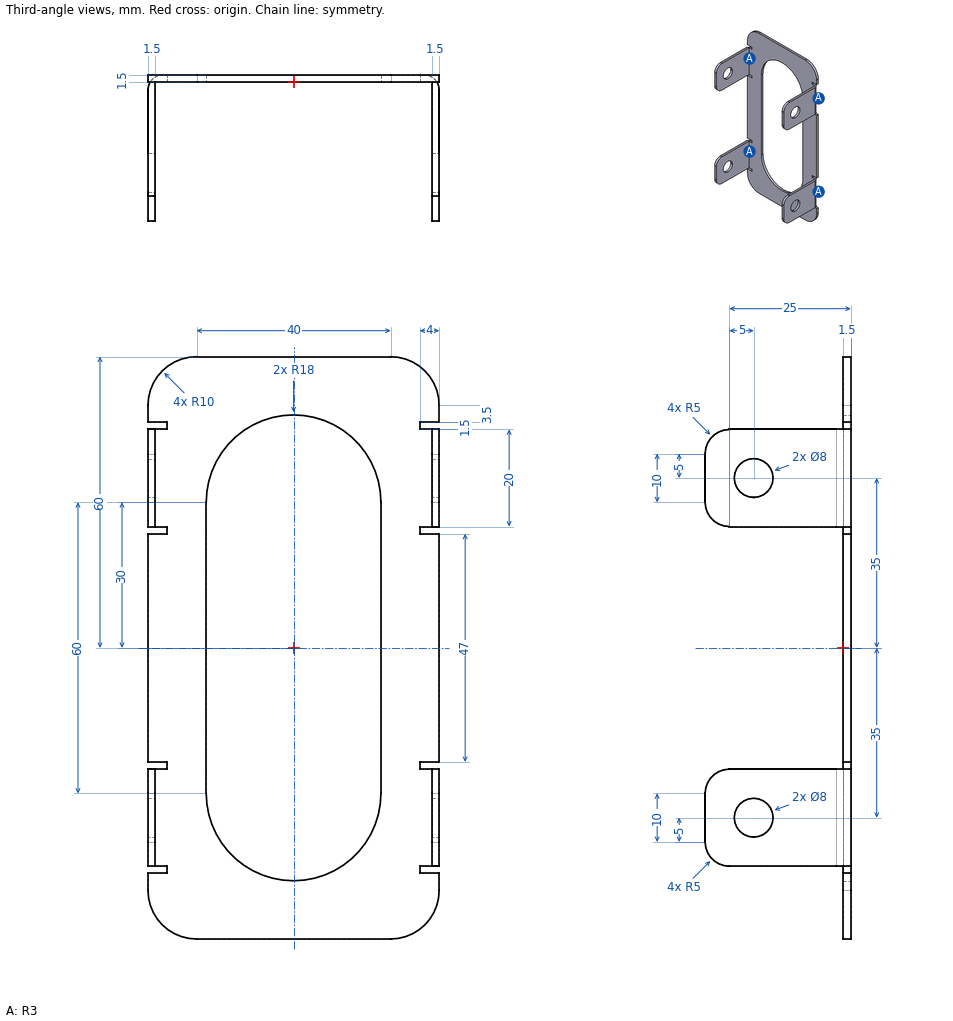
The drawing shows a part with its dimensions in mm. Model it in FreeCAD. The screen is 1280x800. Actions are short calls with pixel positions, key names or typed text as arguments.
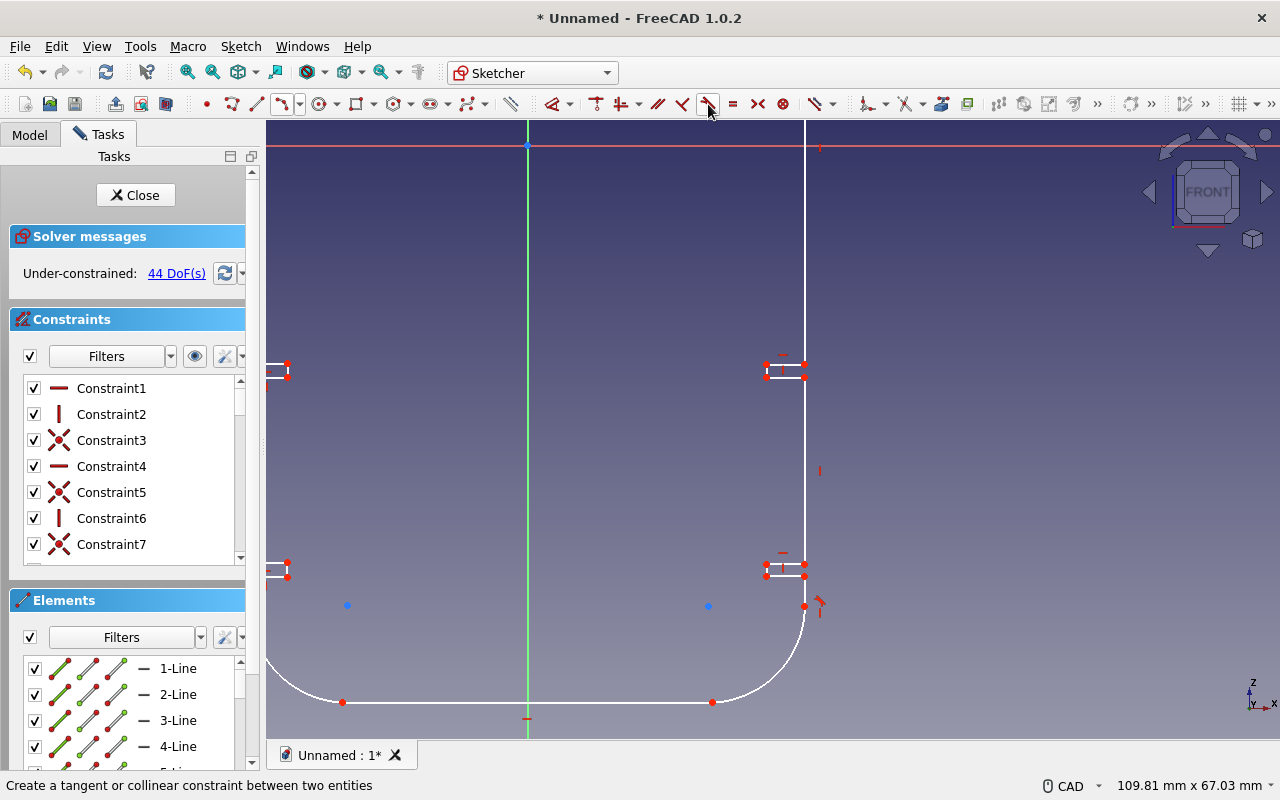
click(602, 703)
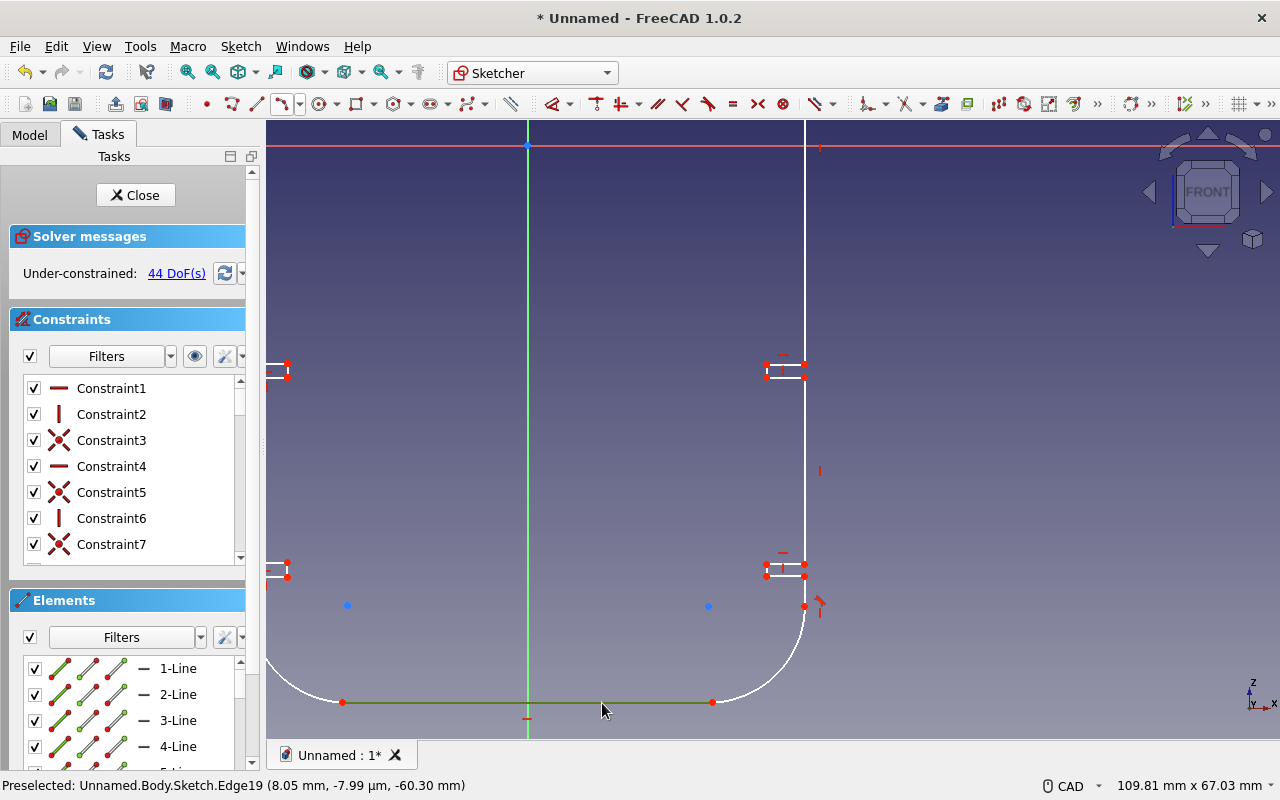
click(755, 691)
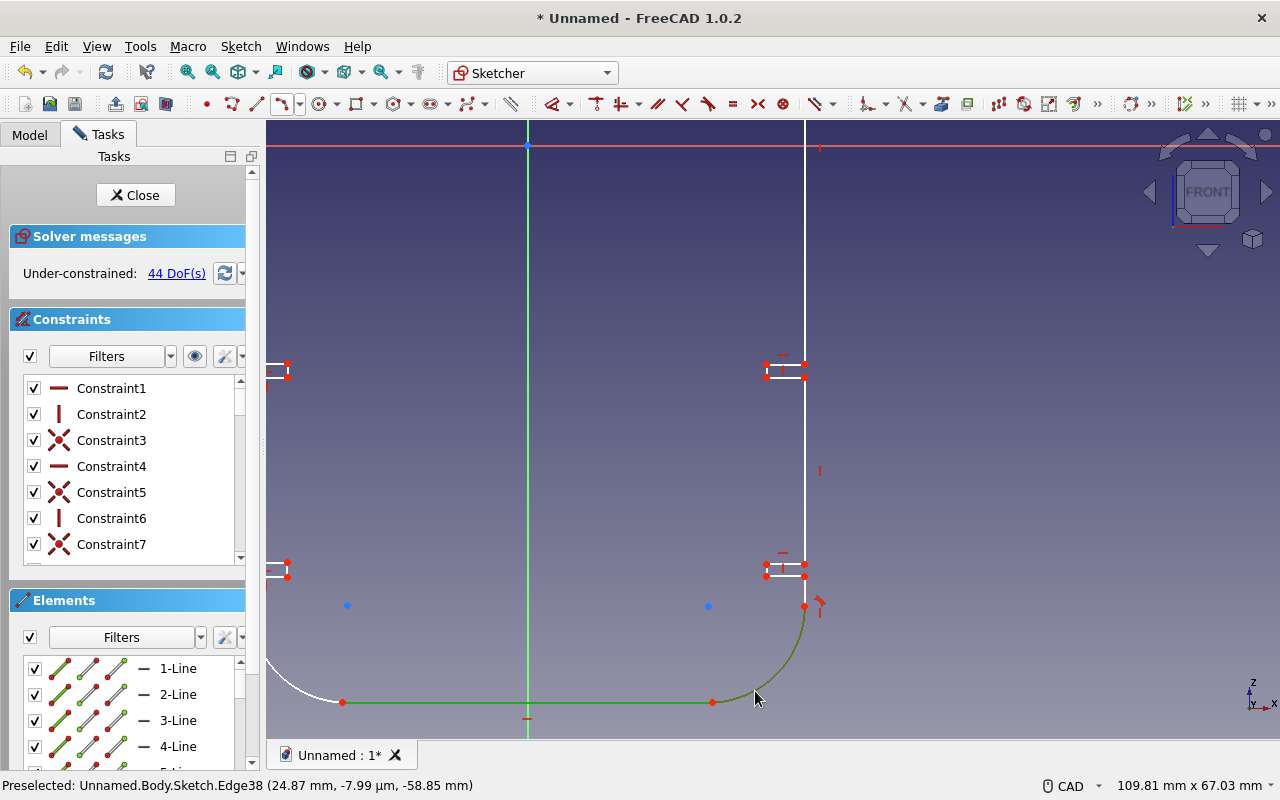
click(708, 104)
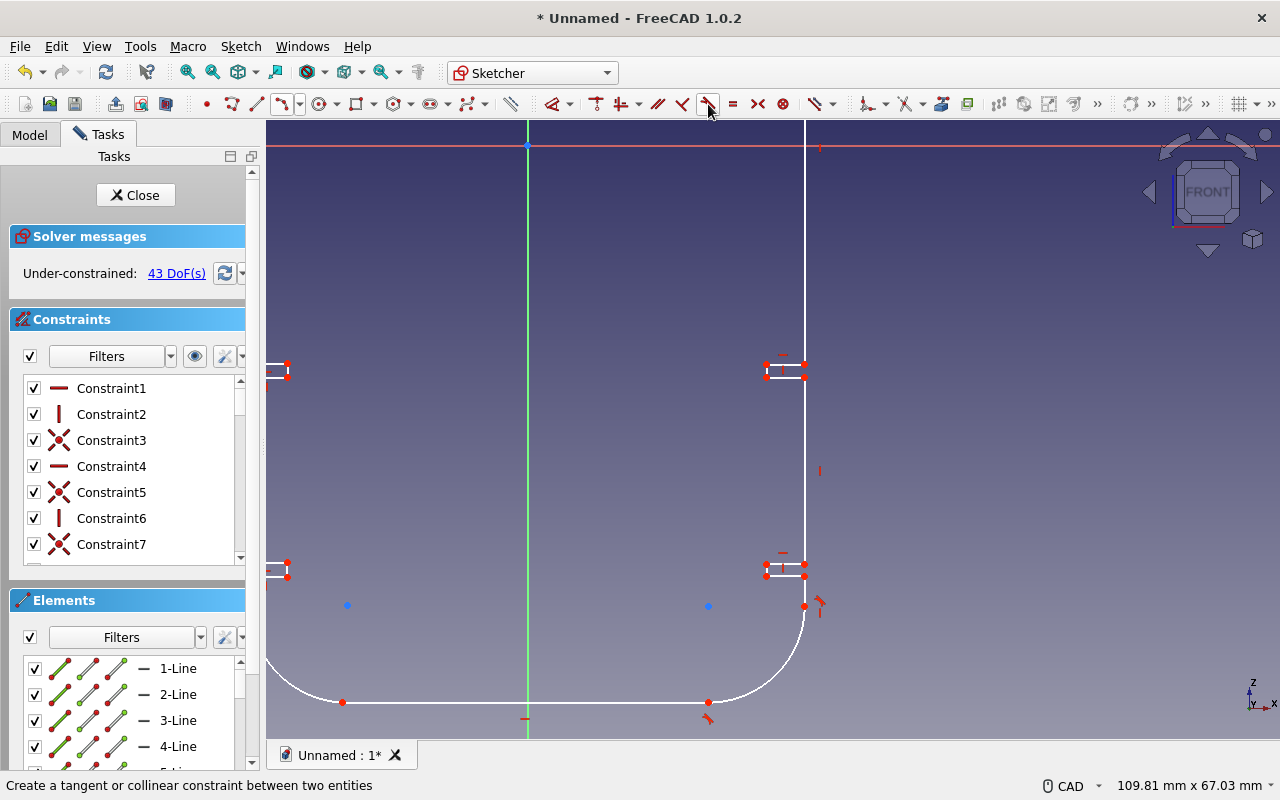
click(599, 703)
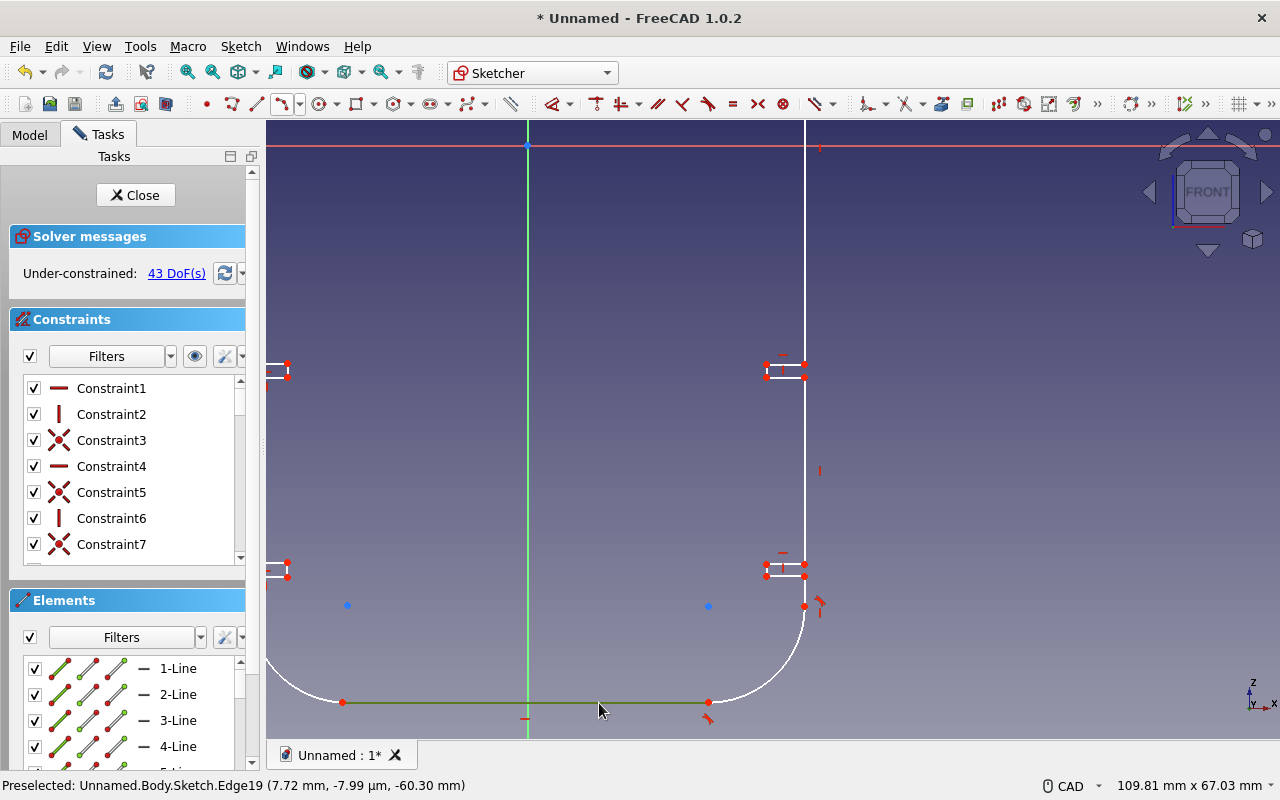
click(302, 691)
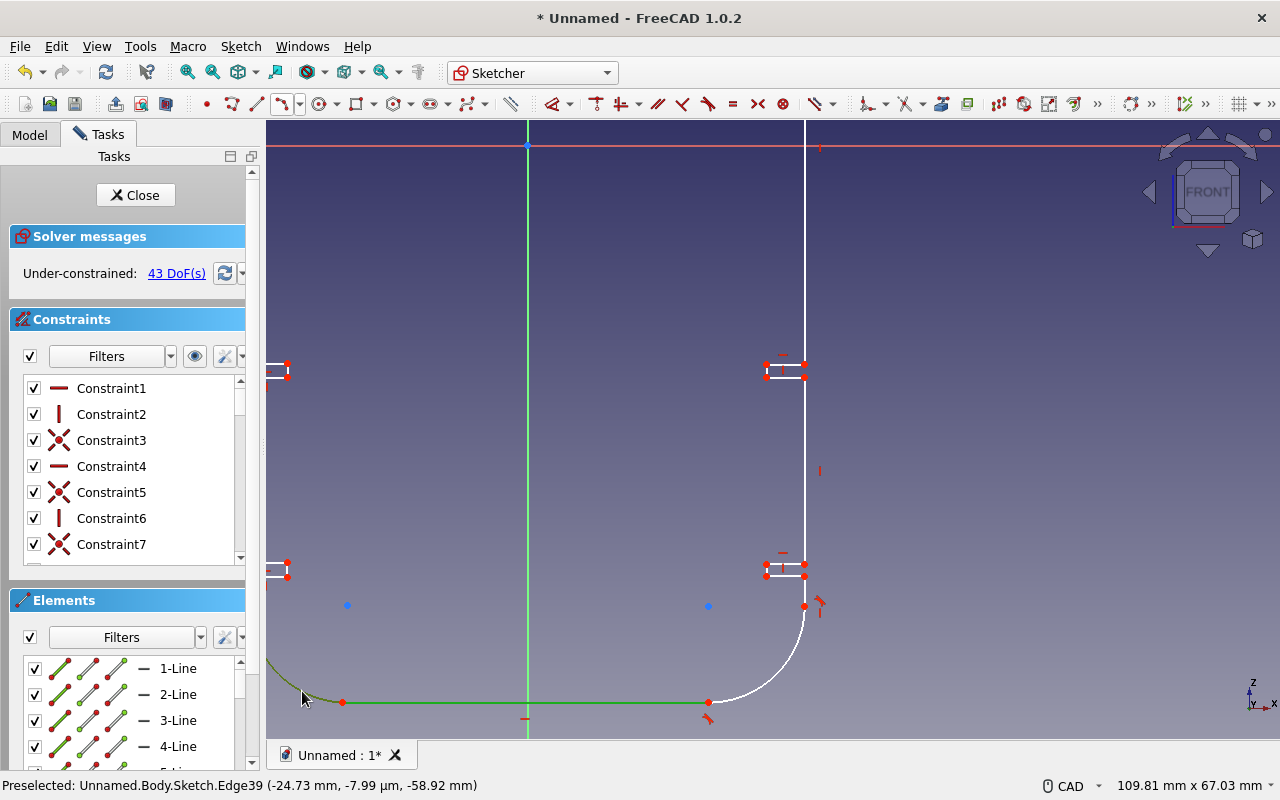
click(708, 104)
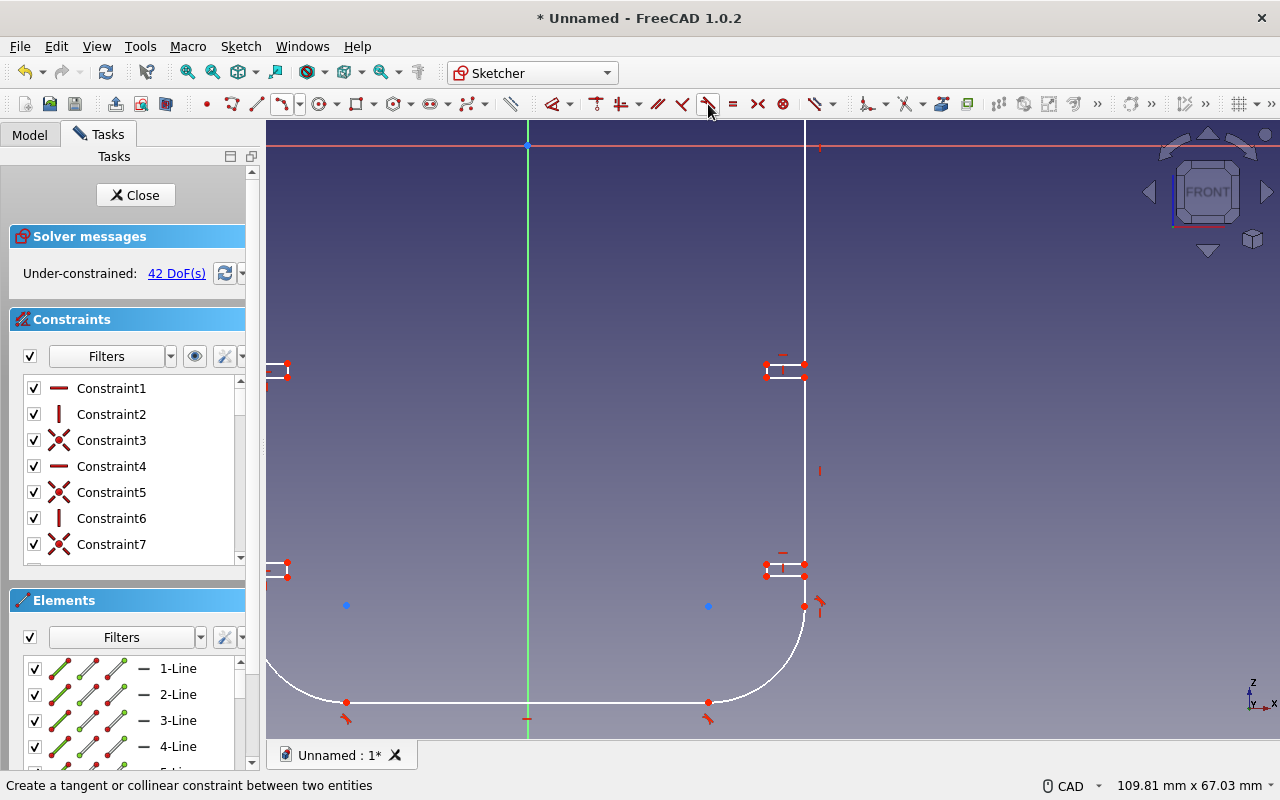
scroll(807, 595, down, 5)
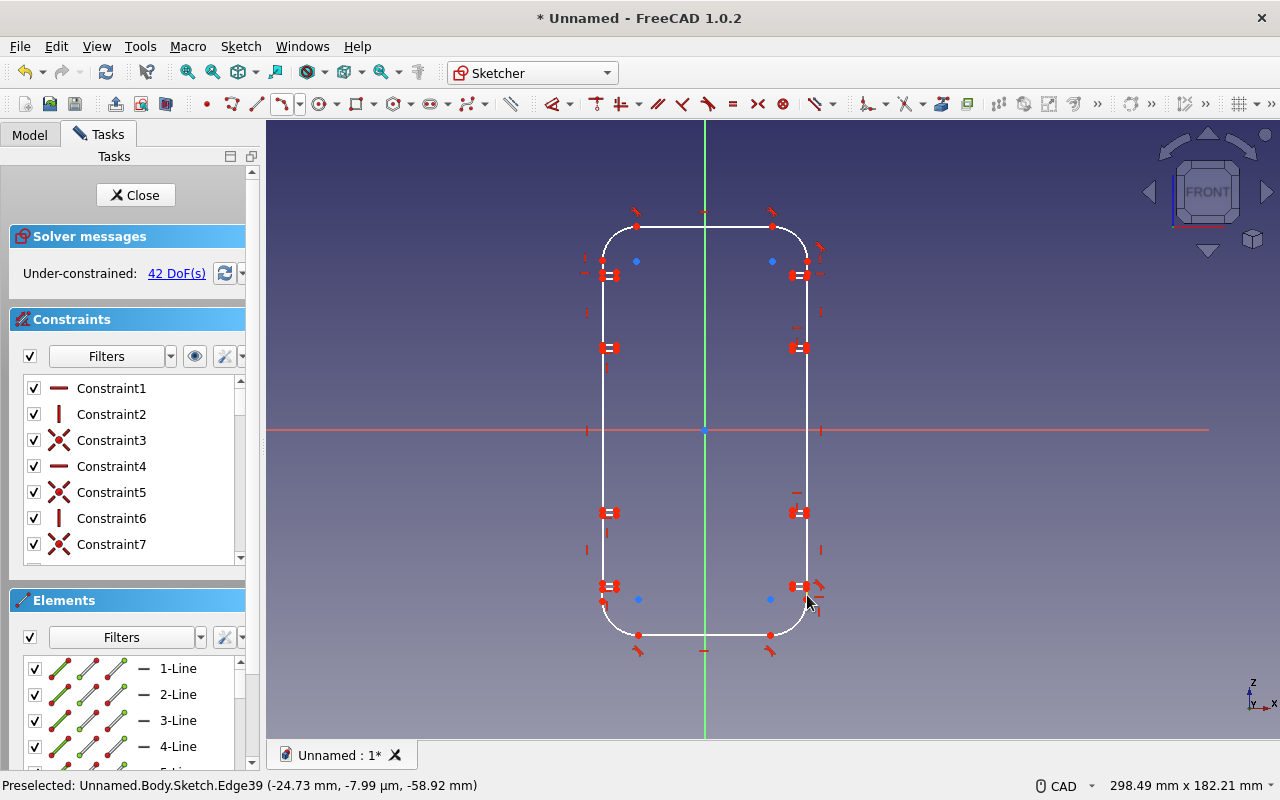
scroll(602, 597, up, 7)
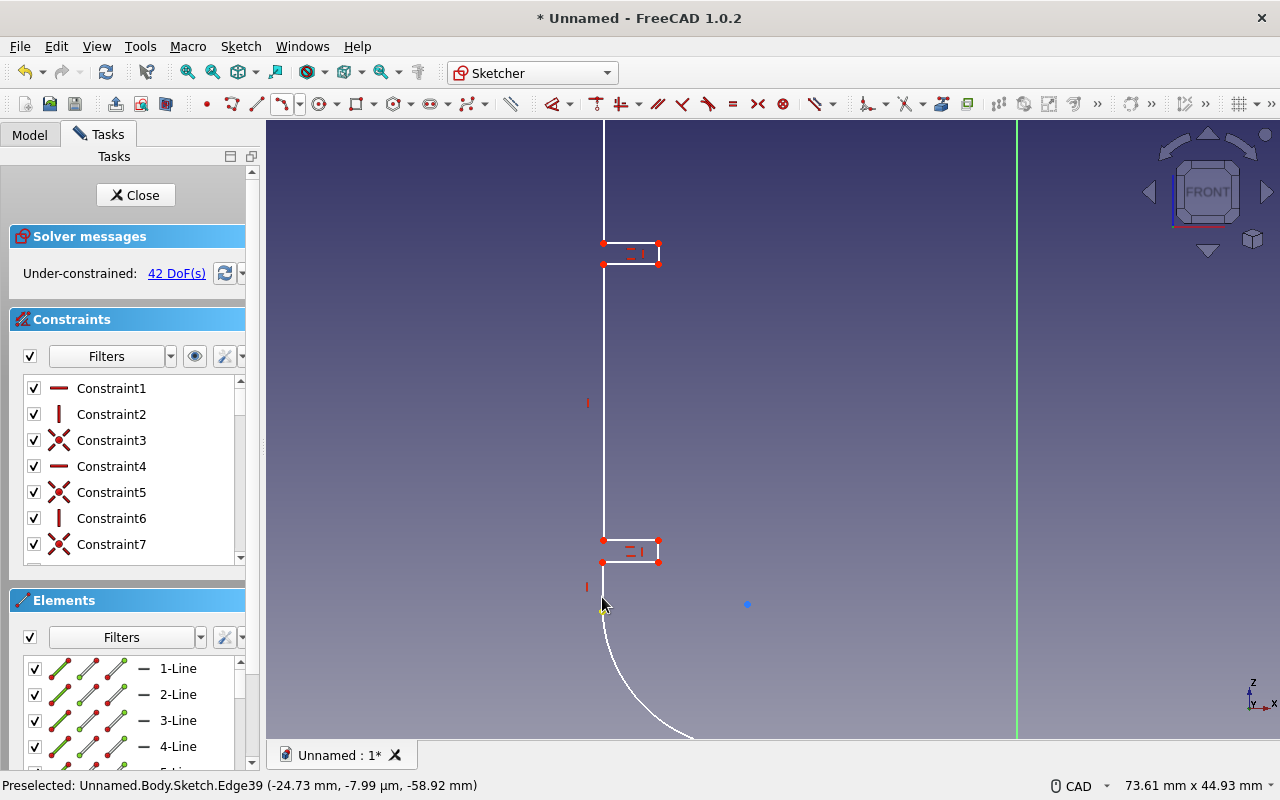
click(603, 597)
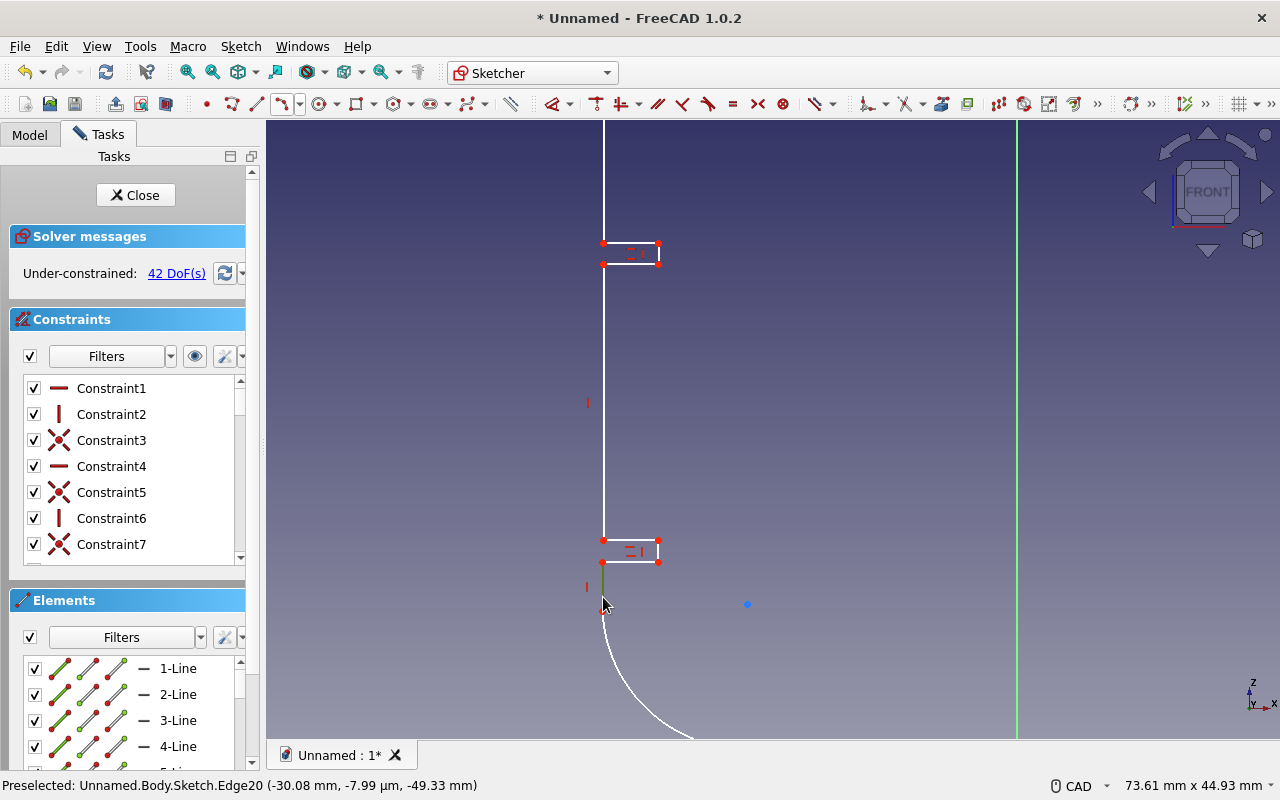
scroll(602, 597, down, 7)